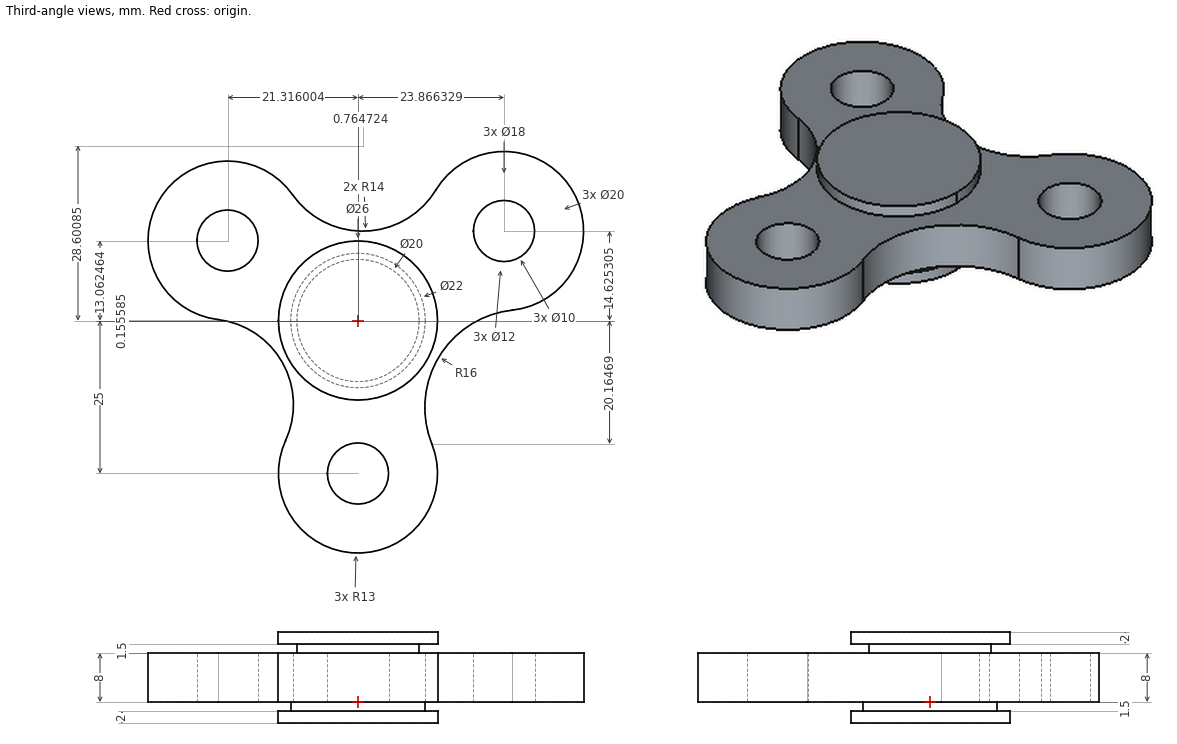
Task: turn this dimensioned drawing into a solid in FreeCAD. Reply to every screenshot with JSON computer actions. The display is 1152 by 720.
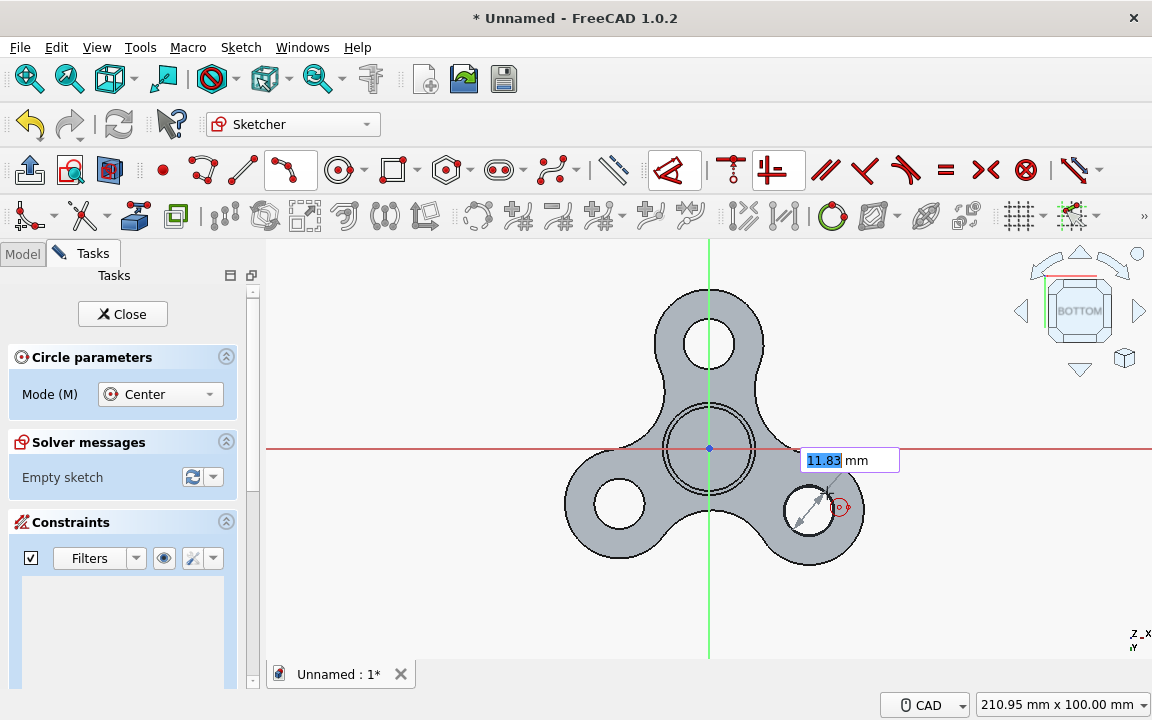
{"action": "type", "text": "12"}
{"action": "key", "text": "Return"}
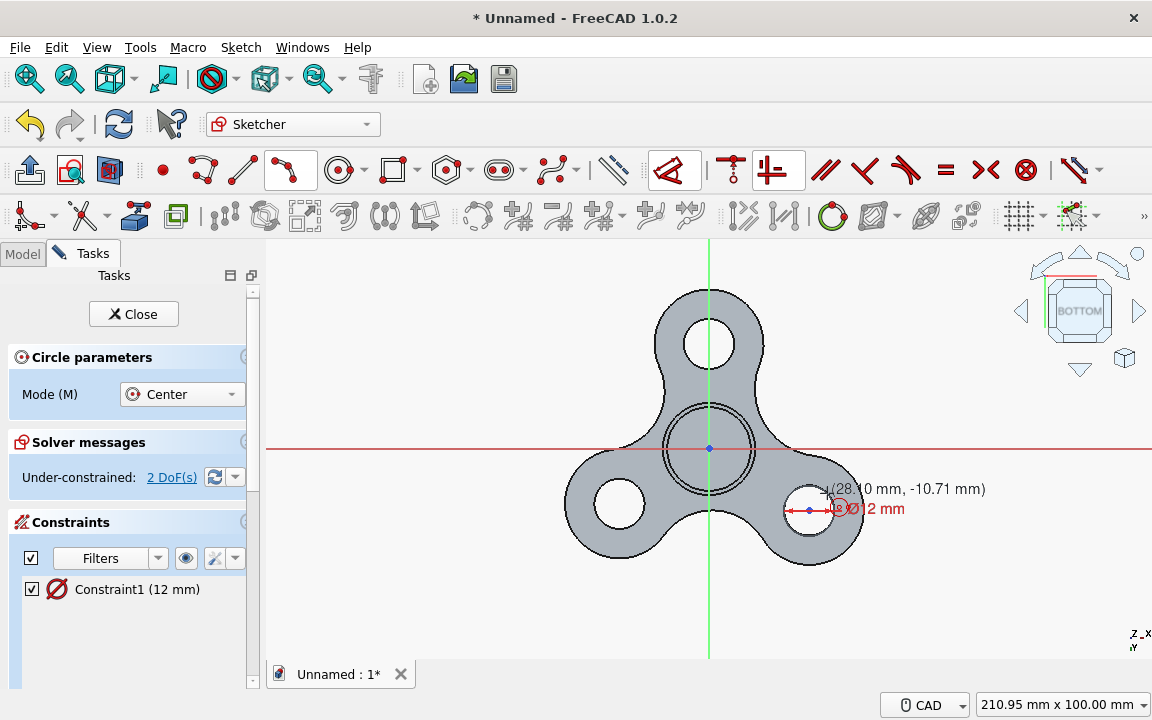
{"action": "left_click", "coordinate": [619, 504]}
{"action": "mouse_move", "coordinate": [637, 486]}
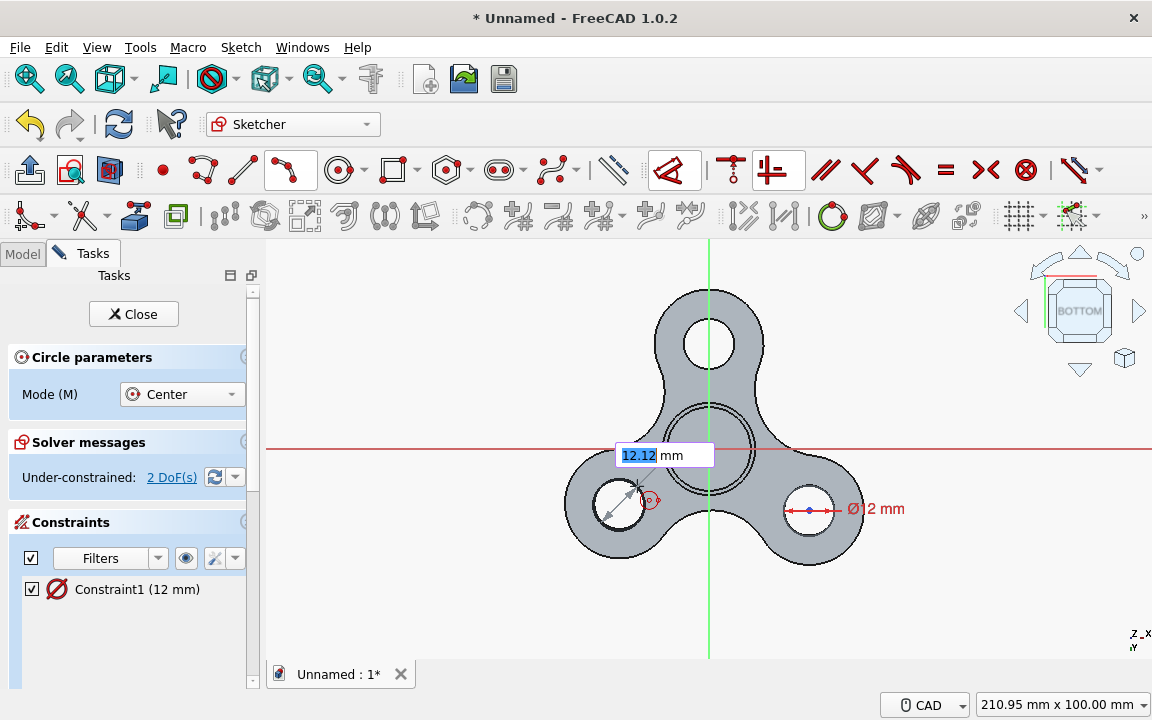
{"action": "type", "text": "12"}
{"action": "key", "text": "Return"}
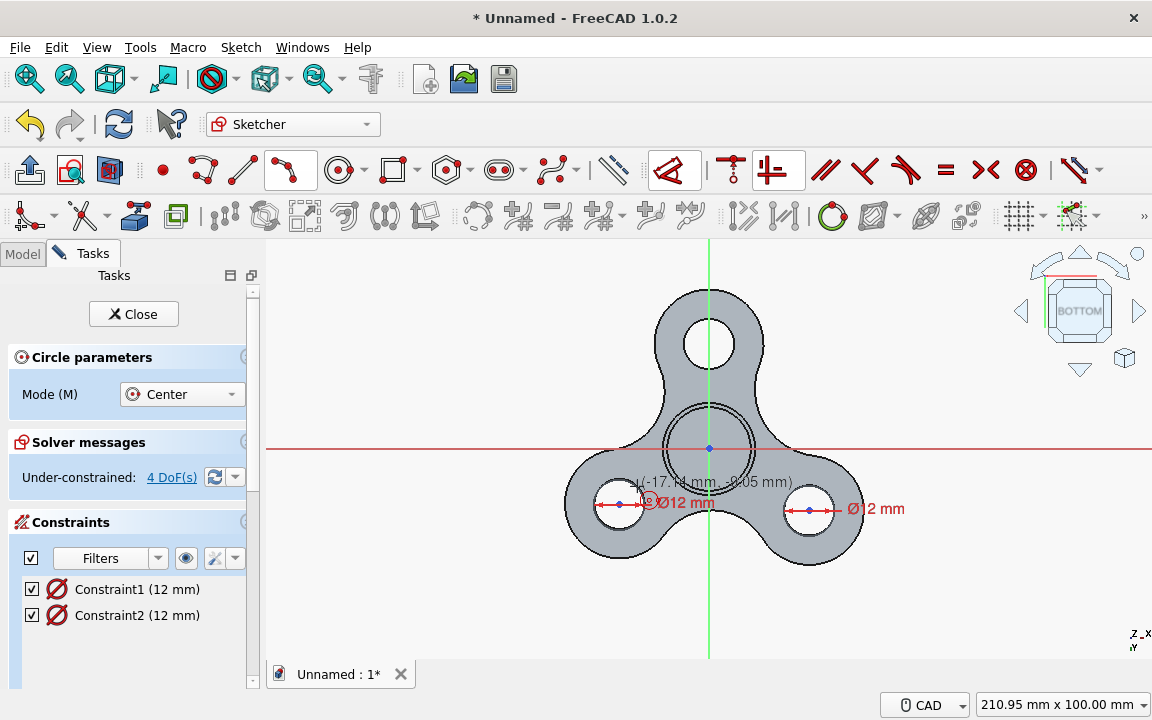
{"action": "left_click", "coordinate": [709, 344]}
{"action": "mouse_move", "coordinate": [727, 326]}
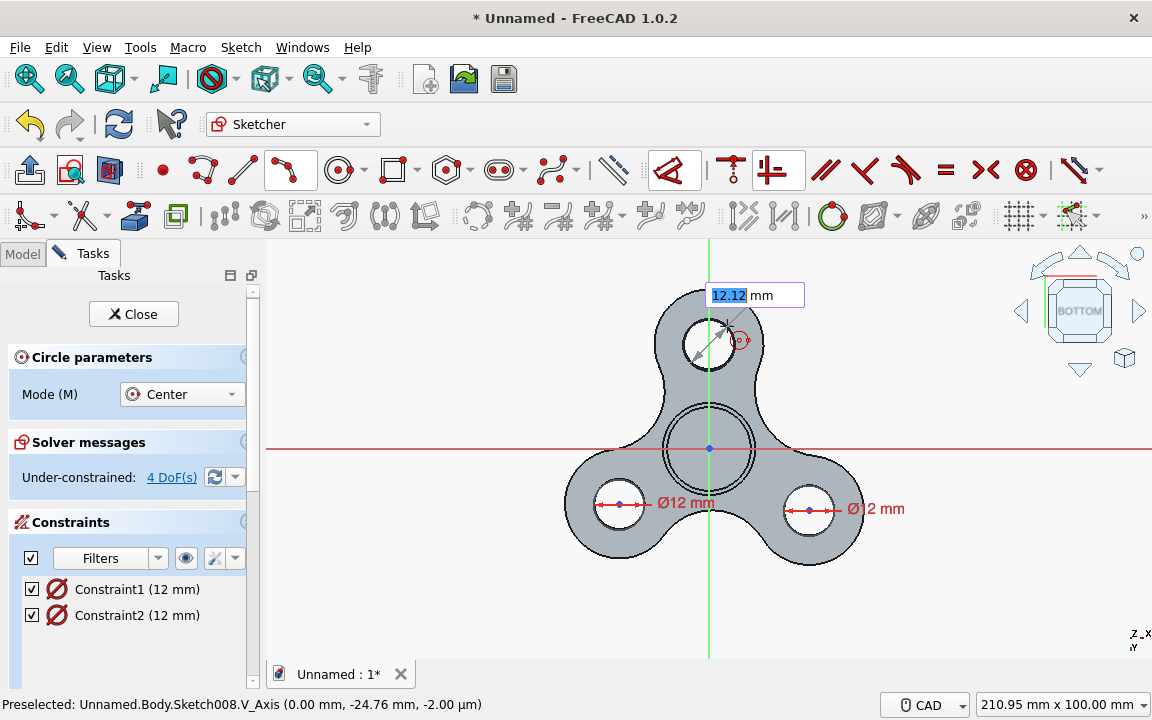
{"action": "type", "text": "12"}
{"action": "key", "text": "Return"}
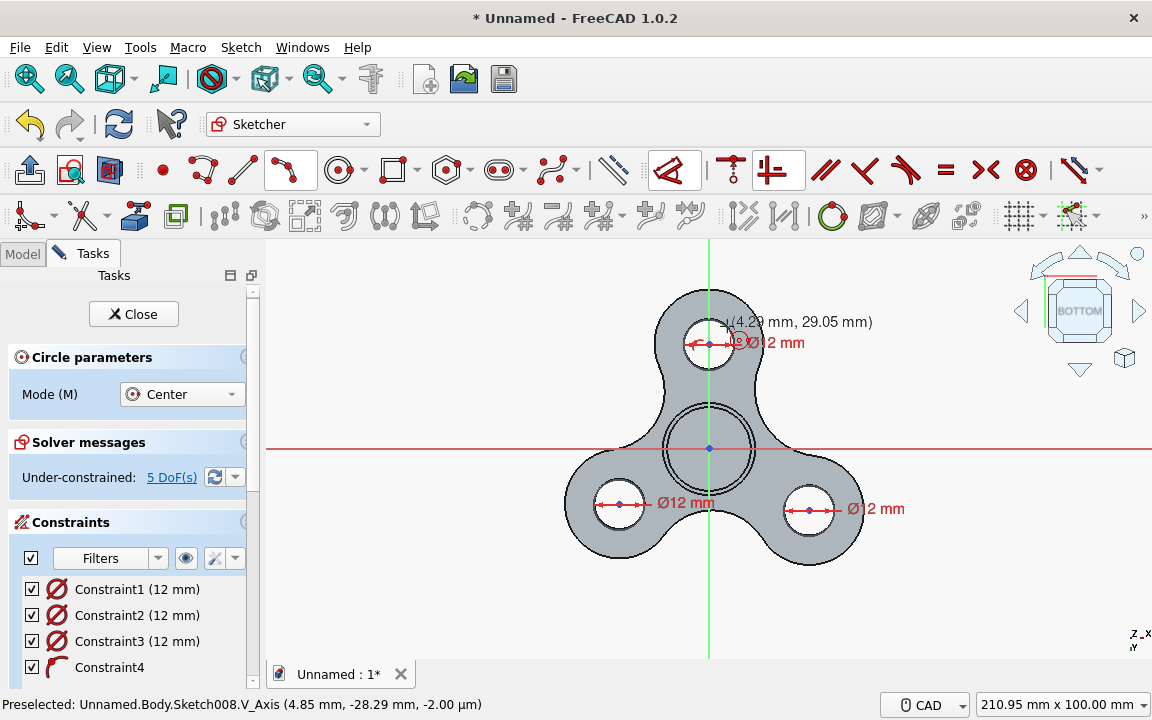
{"action": "left_click", "coordinate": [809, 511]}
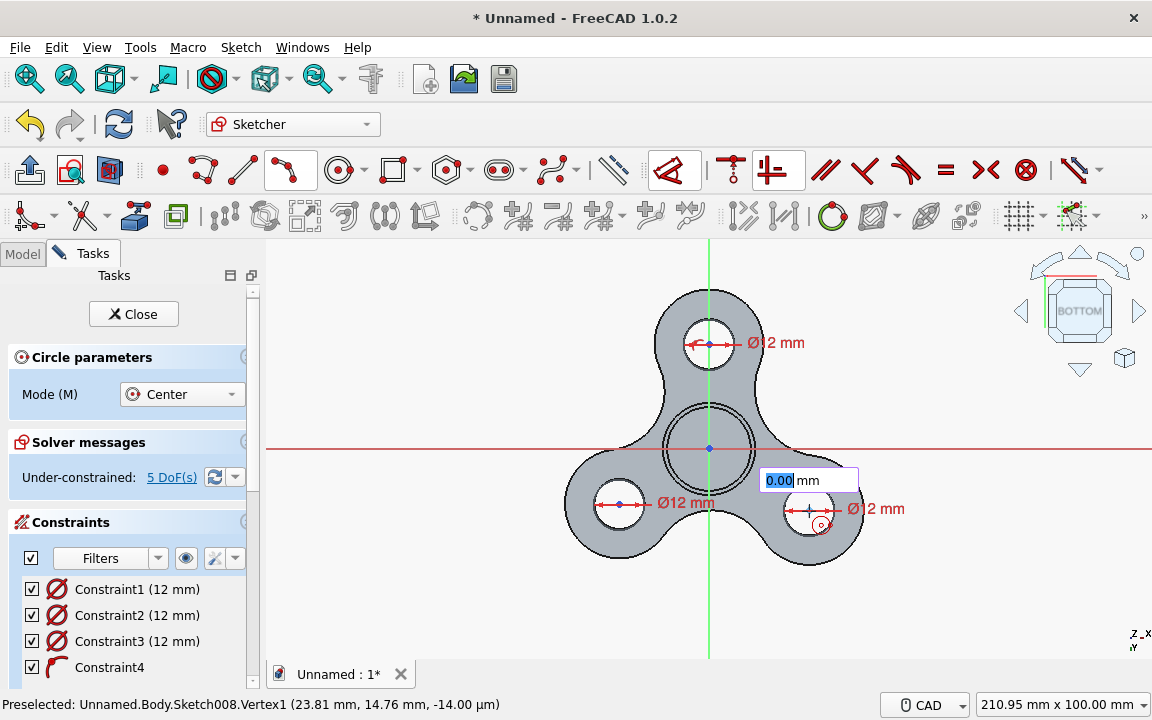
{"action": "scroll", "coordinate": [829, 503], "scroll_direction": "up", "scroll_amount": 7}
{"action": "mouse_move", "coordinate": [827, 502]}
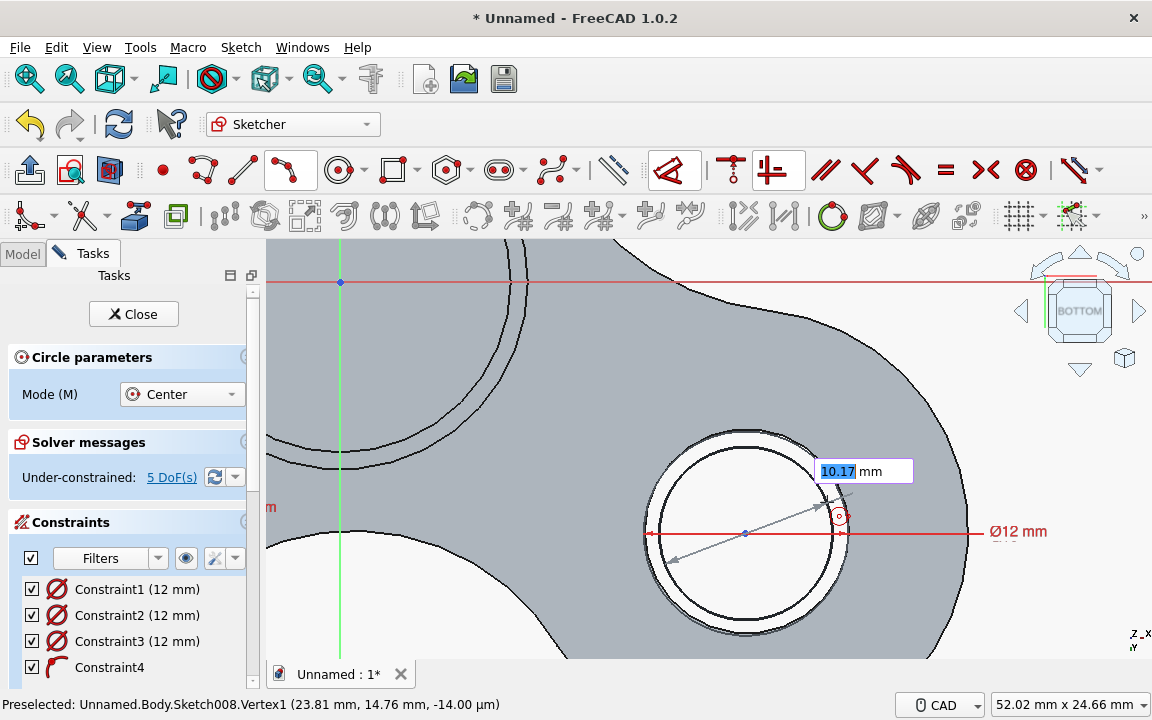
{"action": "type", "text": "10"}
{"action": "key", "text": "Return"}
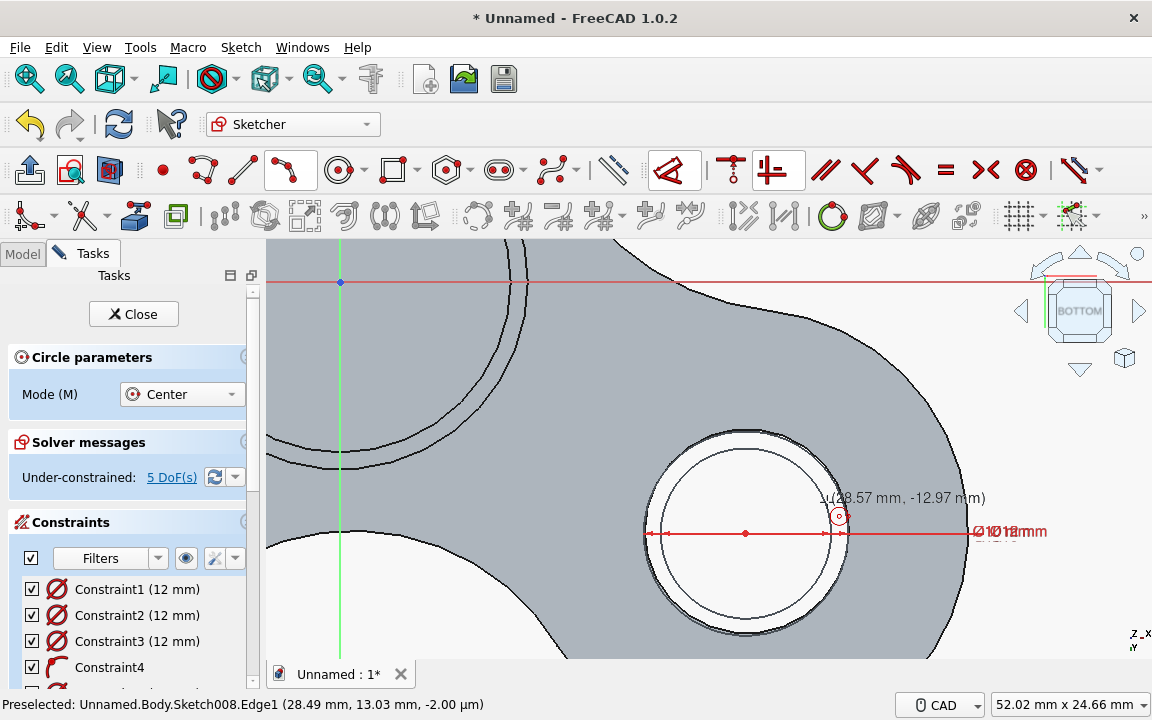
{"action": "scroll", "coordinate": [760, 559], "scroll_direction": "down", "scroll_amount": 6}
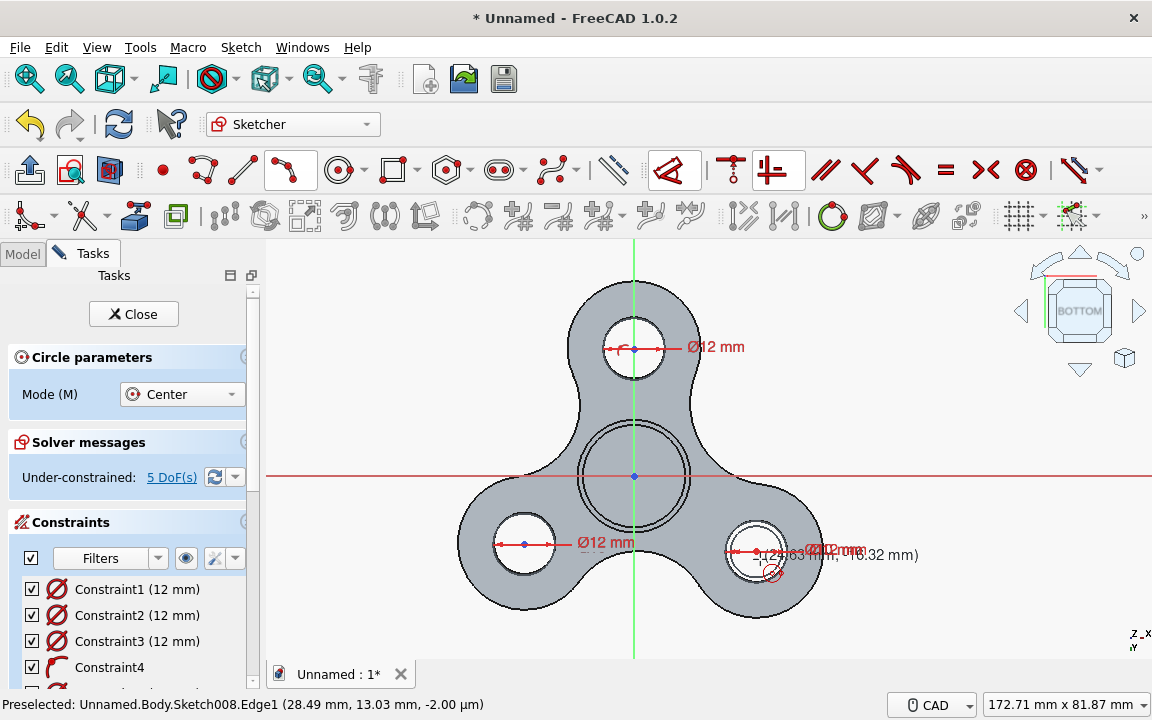
{"action": "left_click", "coordinate": [524, 545]}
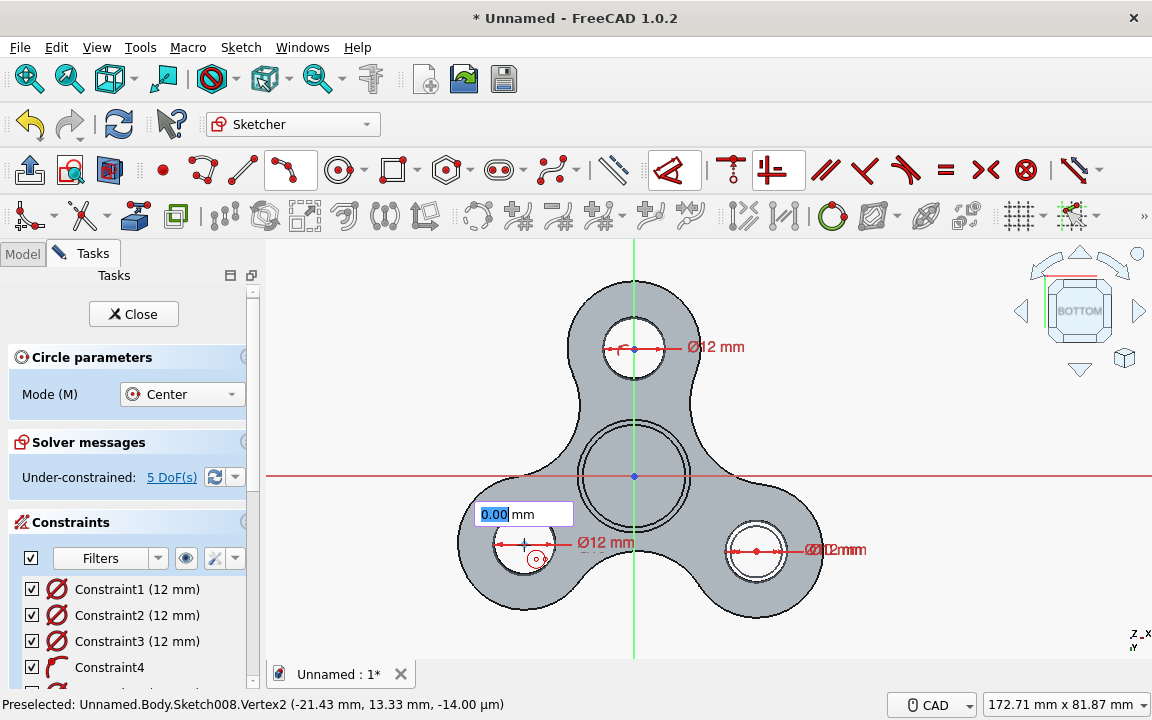
{"action": "scroll", "coordinate": [507, 561], "scroll_direction": "up", "scroll_amount": 6}
{"action": "mouse_move", "coordinate": [505, 560]}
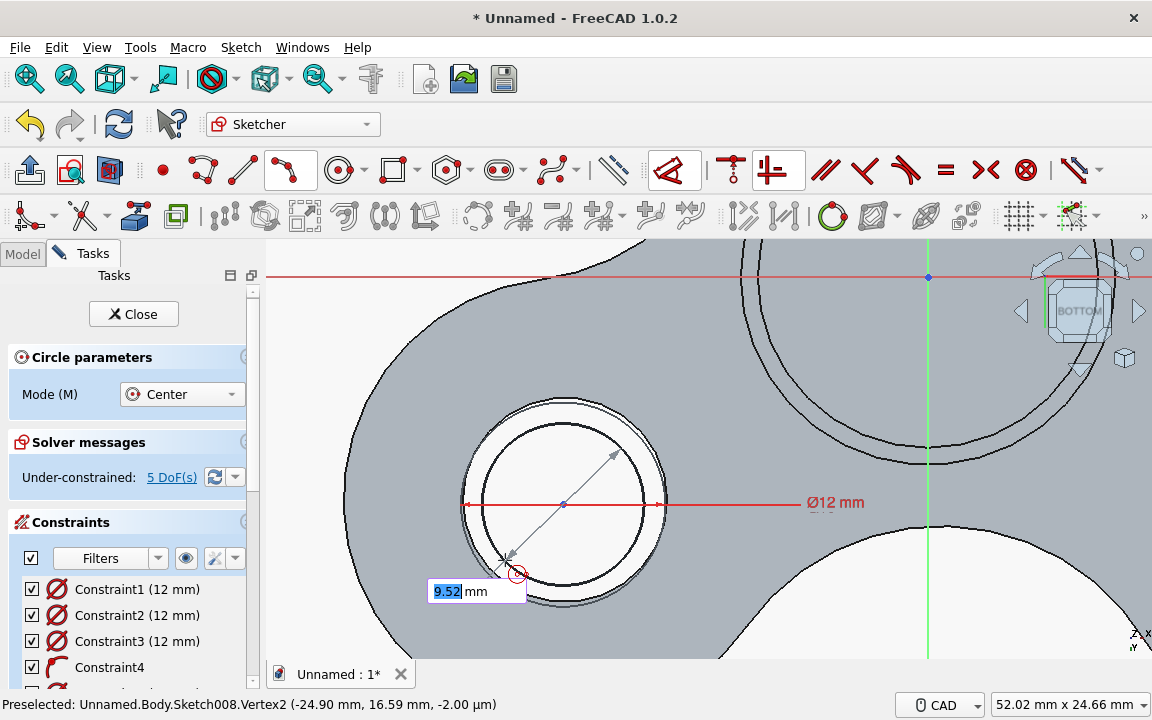
{"action": "type", "text": "10"}
{"action": "key", "text": "Return"}